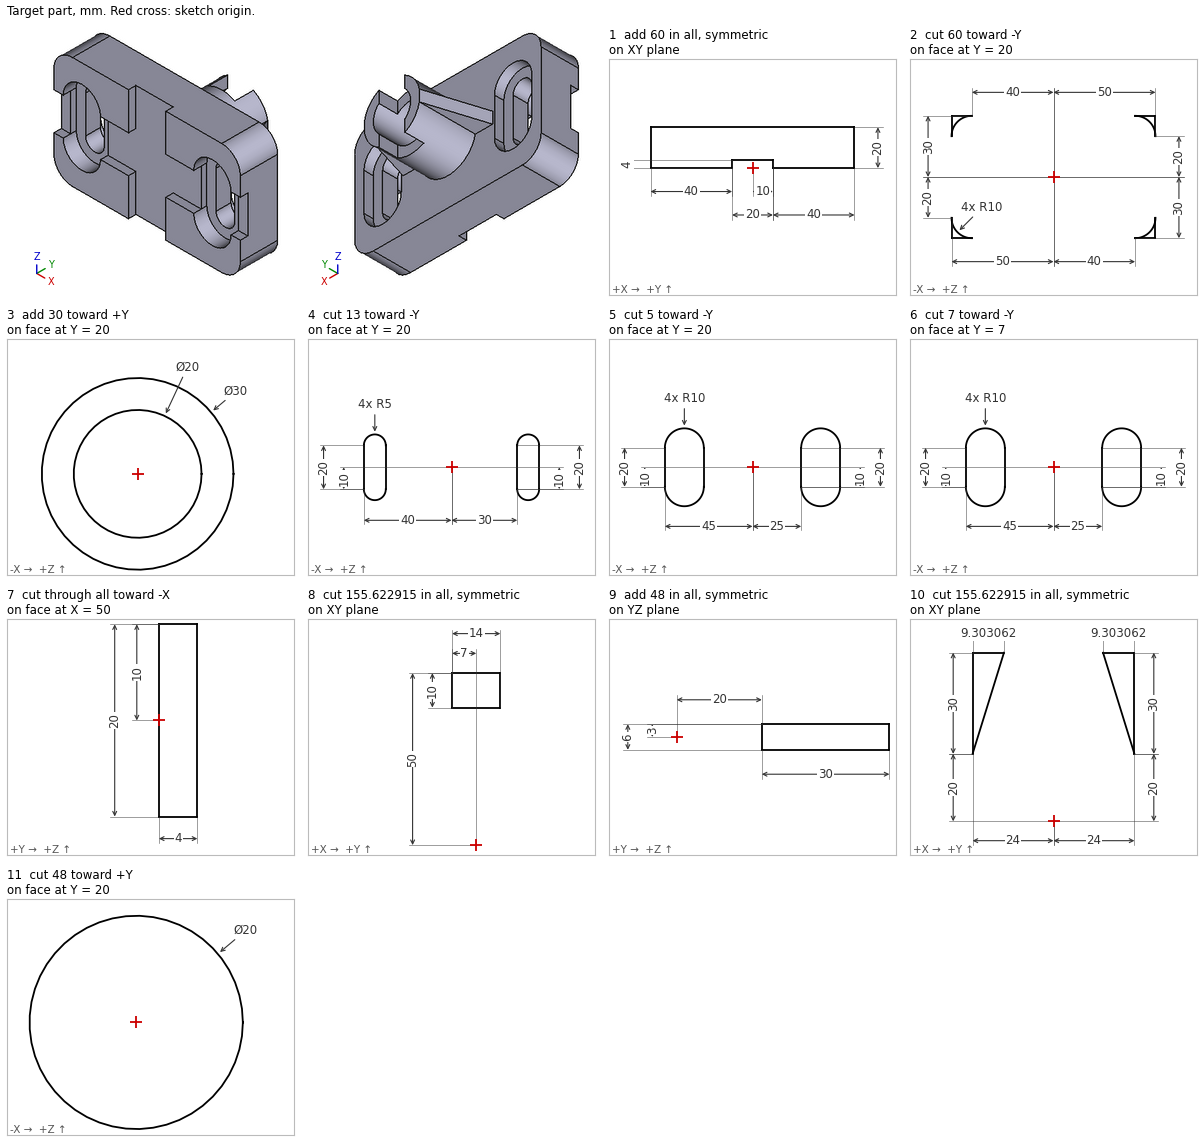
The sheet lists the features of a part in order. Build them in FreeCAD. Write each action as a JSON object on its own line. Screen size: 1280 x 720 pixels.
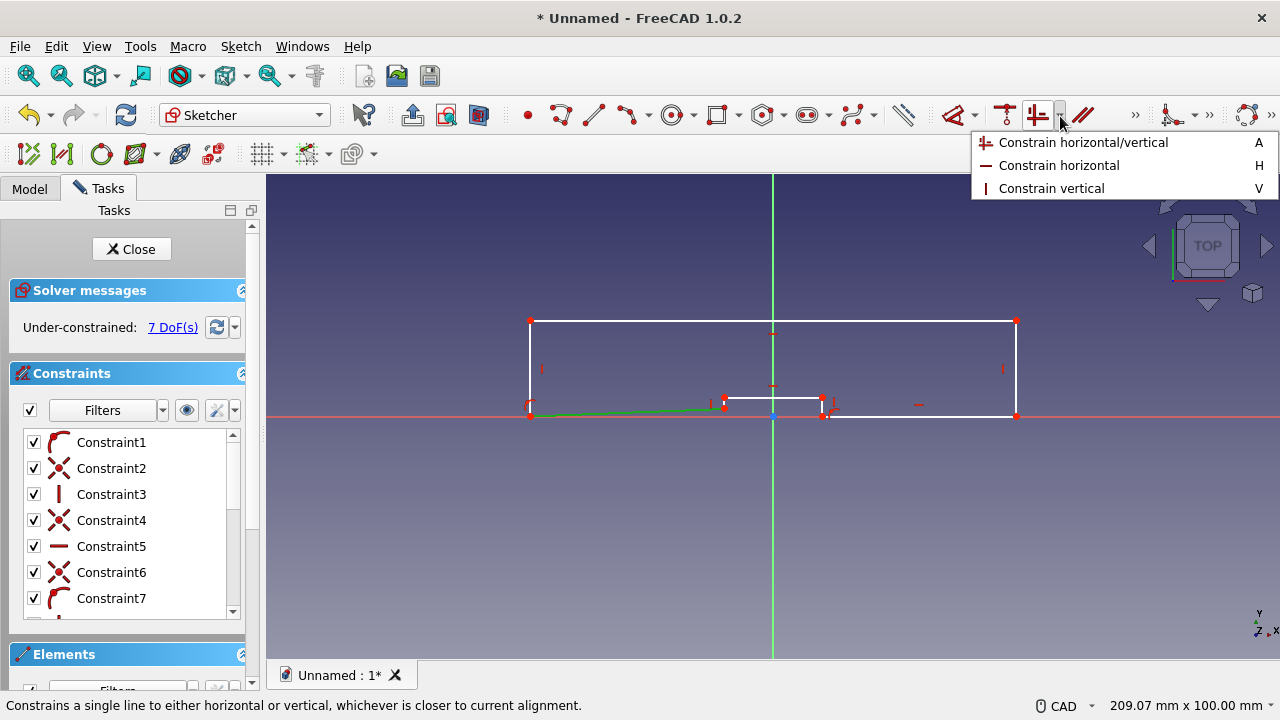
{"action": "left_click", "coordinate": [1125, 166]}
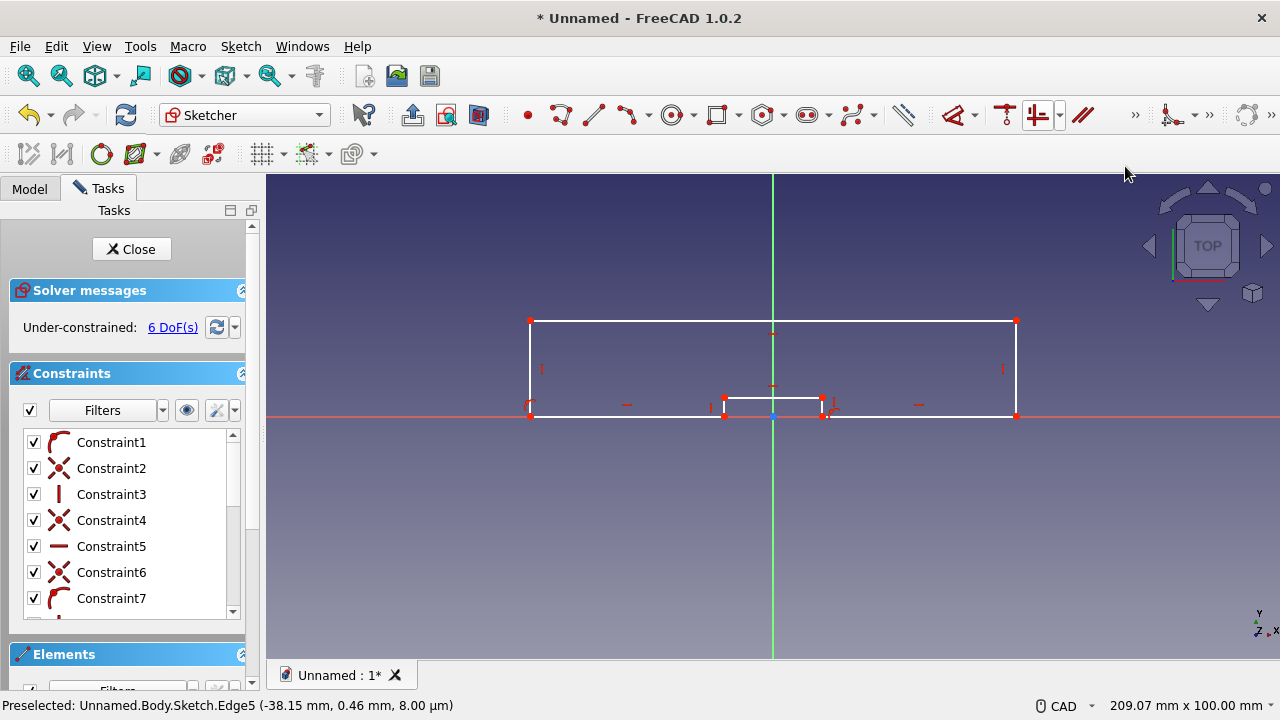
{"action": "scroll", "coordinate": [724, 407], "scroll_direction": "up", "scroll_amount": 4}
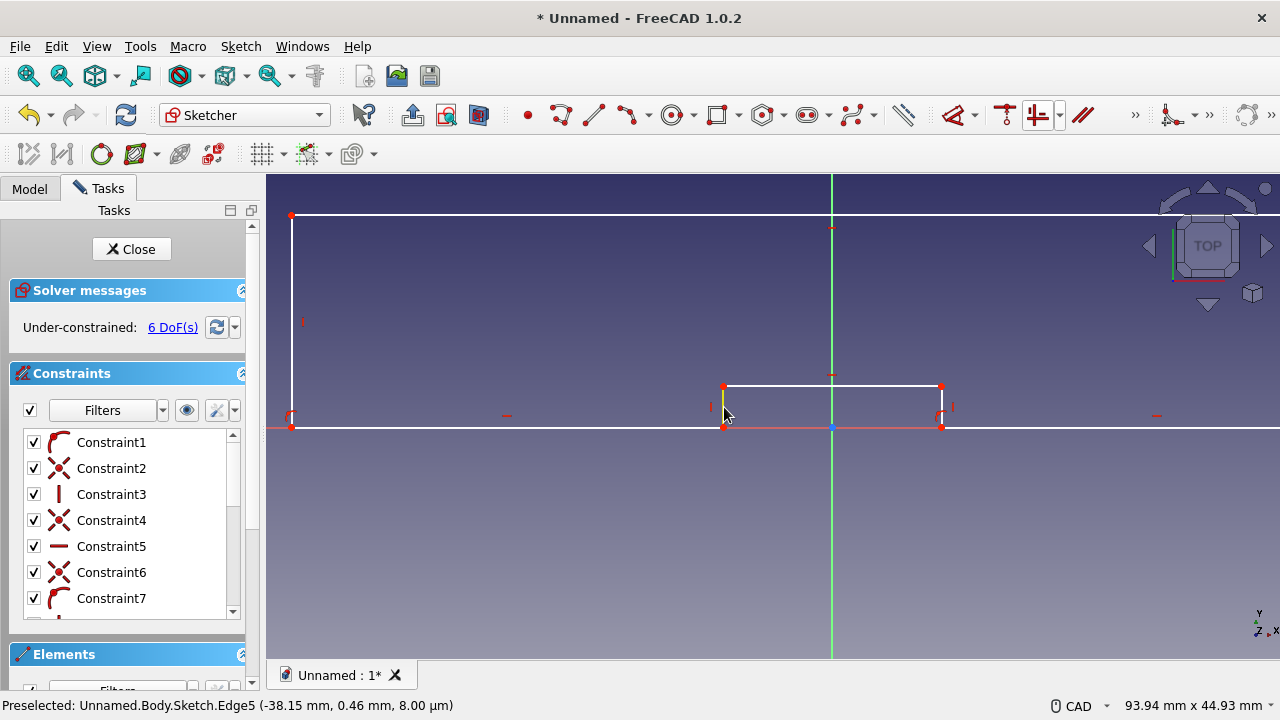
{"action": "left_click", "coordinate": [723, 407]}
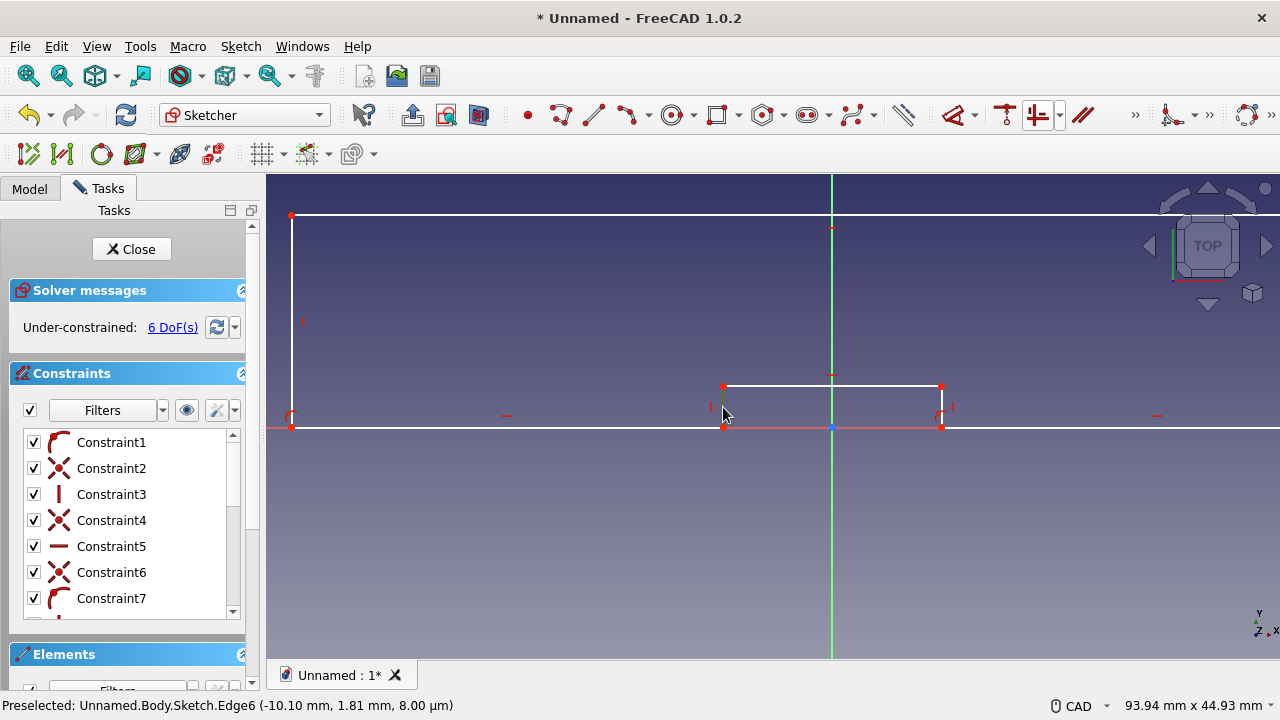
{"action": "key", "text": "i"}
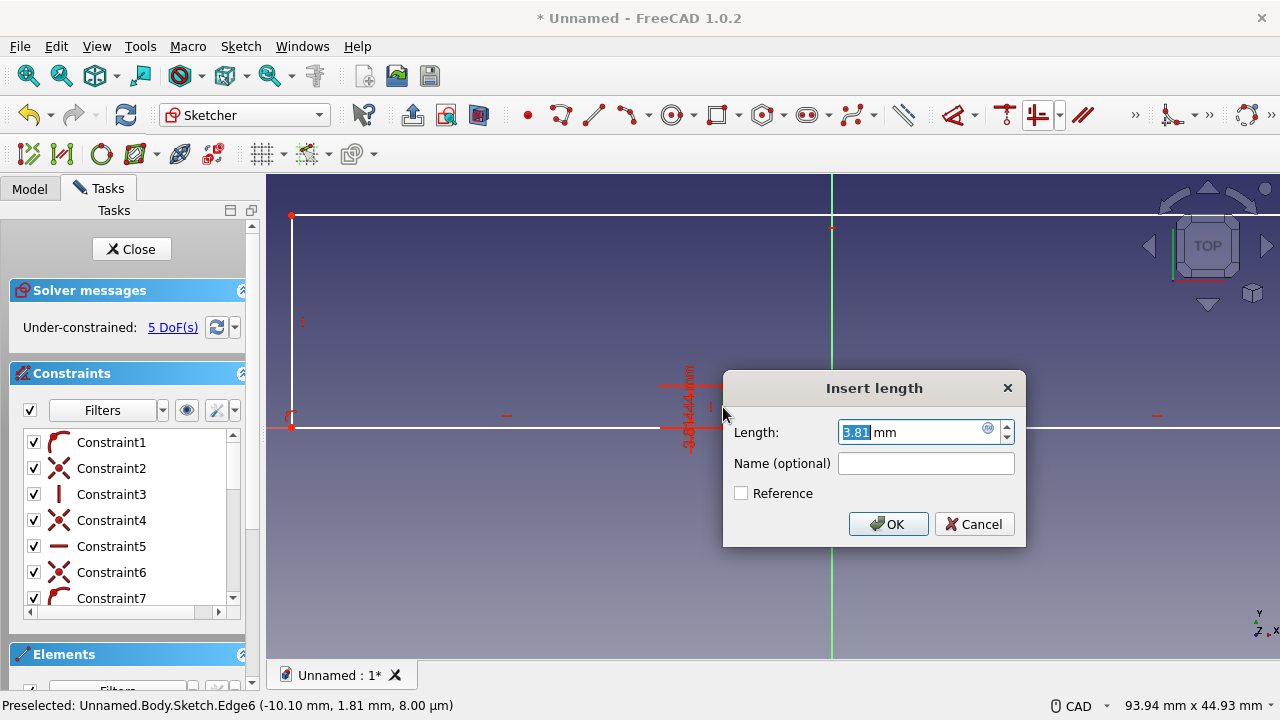
{"action": "type", "text": "4"}
{"action": "key", "text": "Return"}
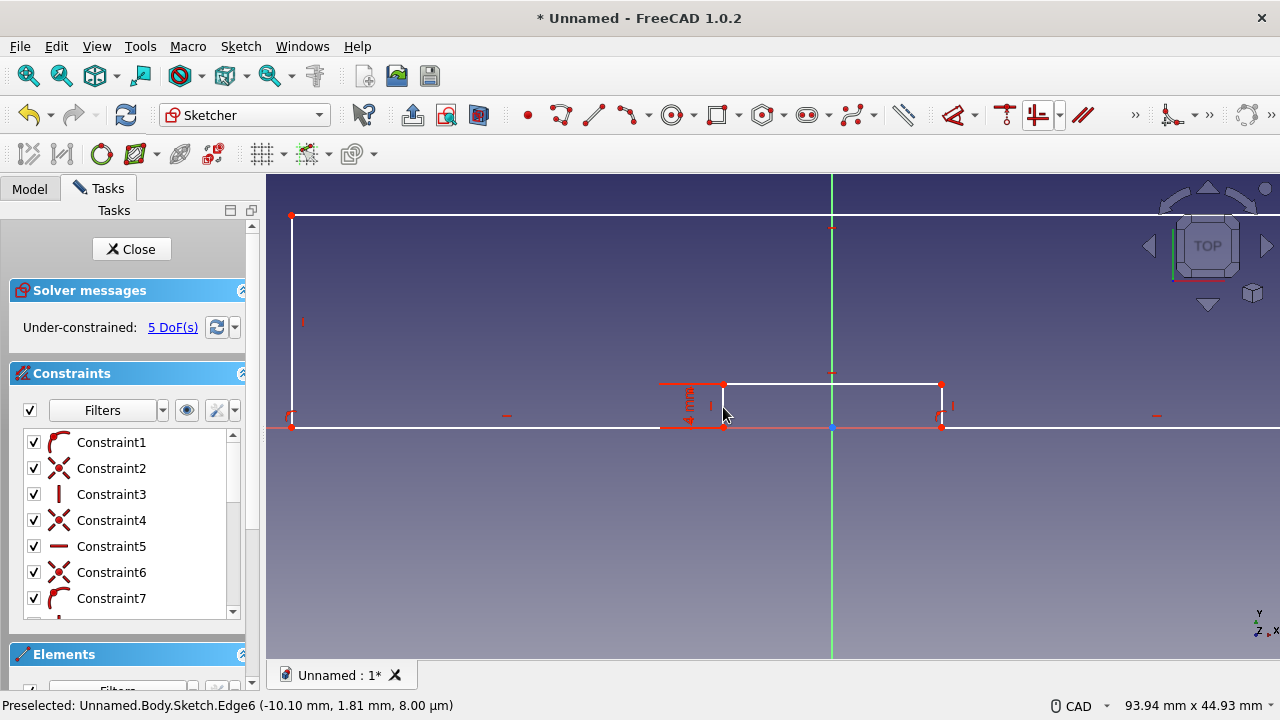
{"action": "left_click", "coordinate": [1071, 428]}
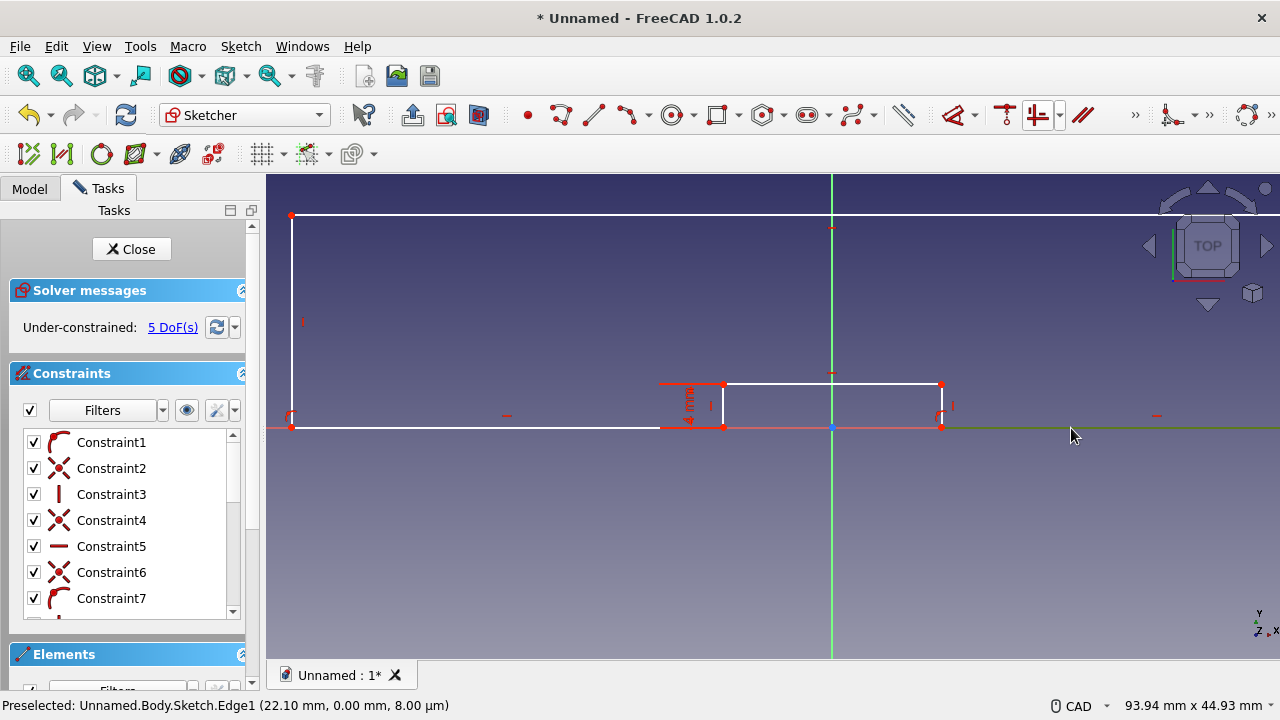
{"action": "left_click", "coordinate": [974, 116]}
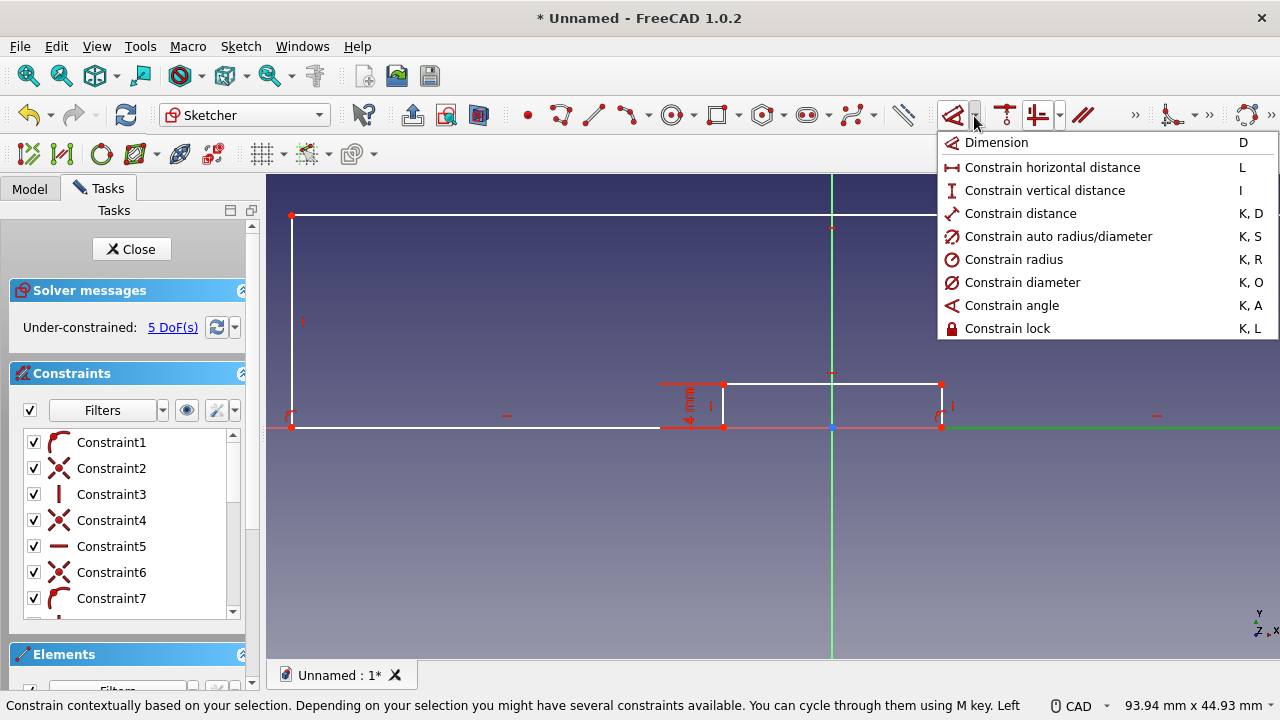
{"action": "left_click", "coordinate": [1108, 168]}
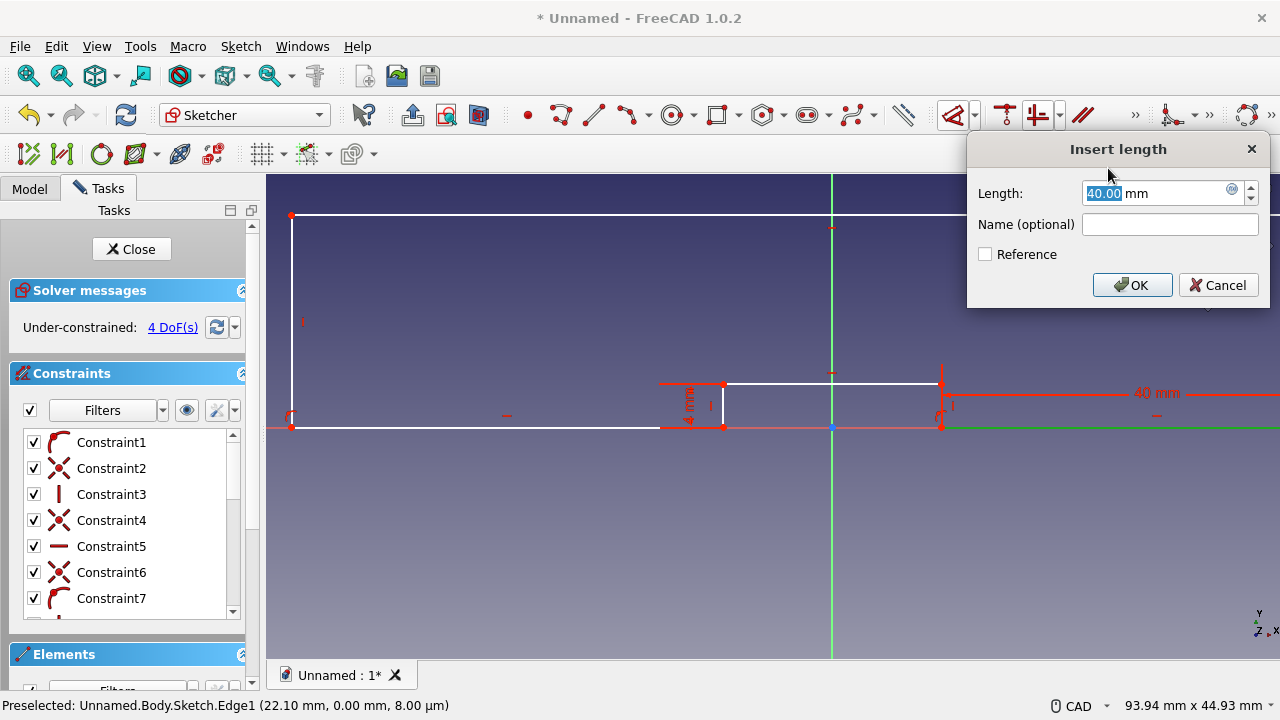
{"action": "type", "text": "40"}
{"action": "key", "text": "Return"}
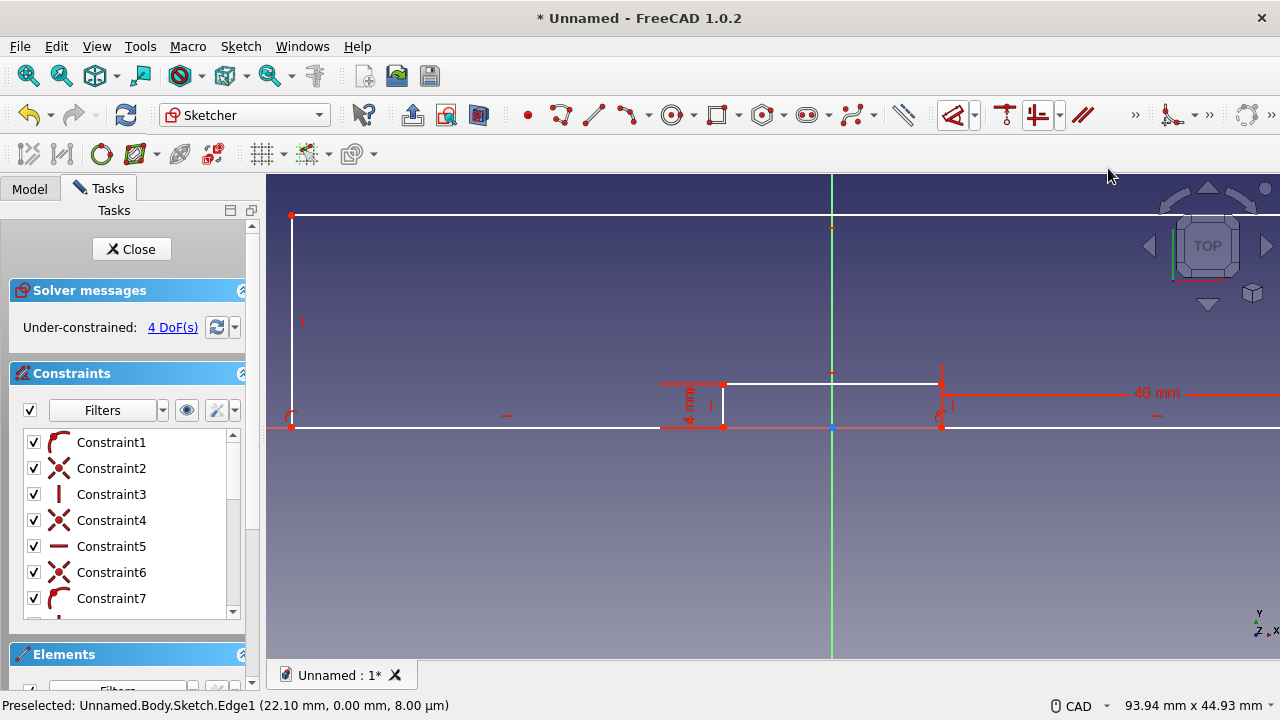
{"action": "scroll", "coordinate": [549, 534], "scroll_direction": "down", "scroll_amount": 3}